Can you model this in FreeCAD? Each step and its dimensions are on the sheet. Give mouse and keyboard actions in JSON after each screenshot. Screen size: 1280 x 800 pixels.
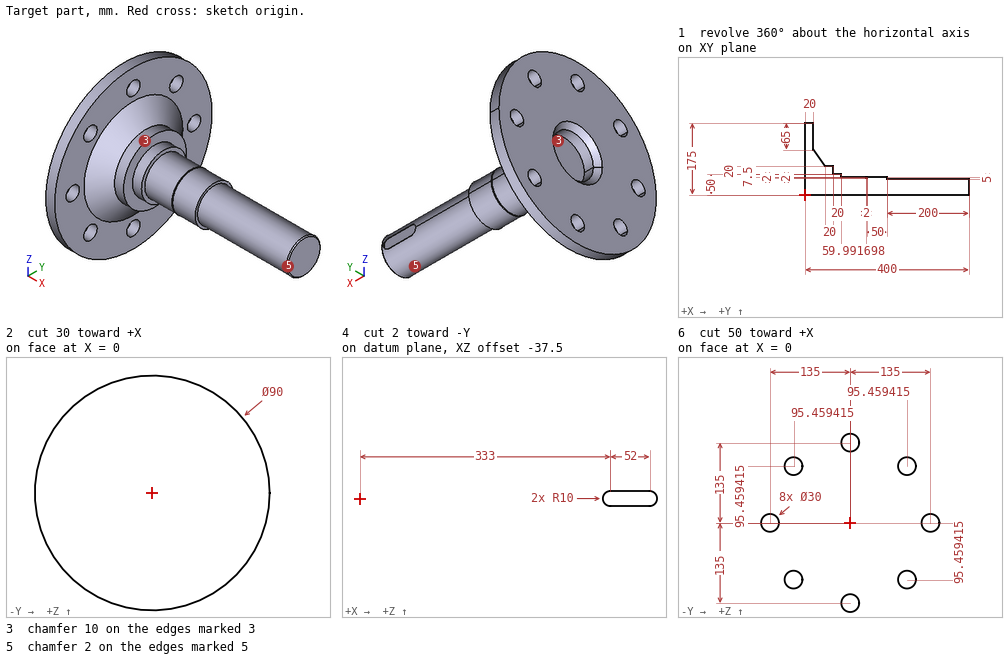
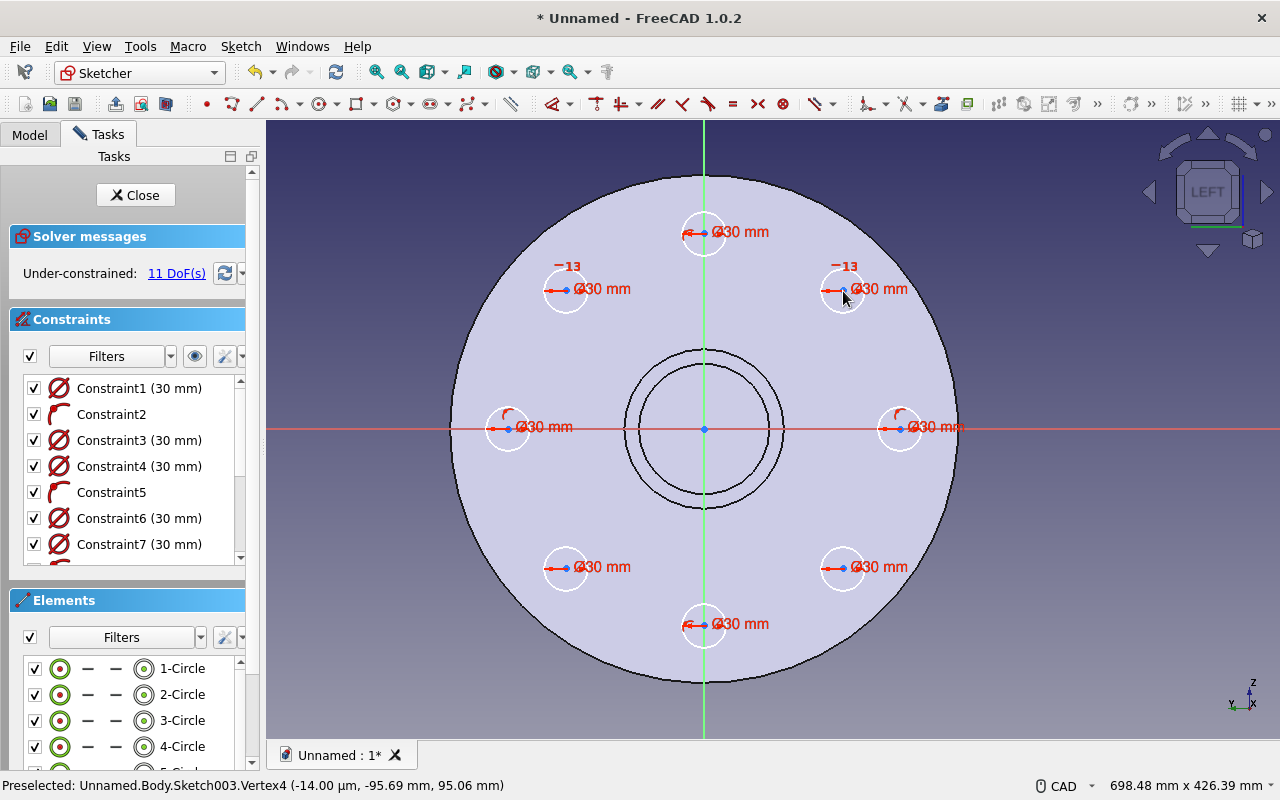
{"action": "left_click", "coordinate": [843, 291]}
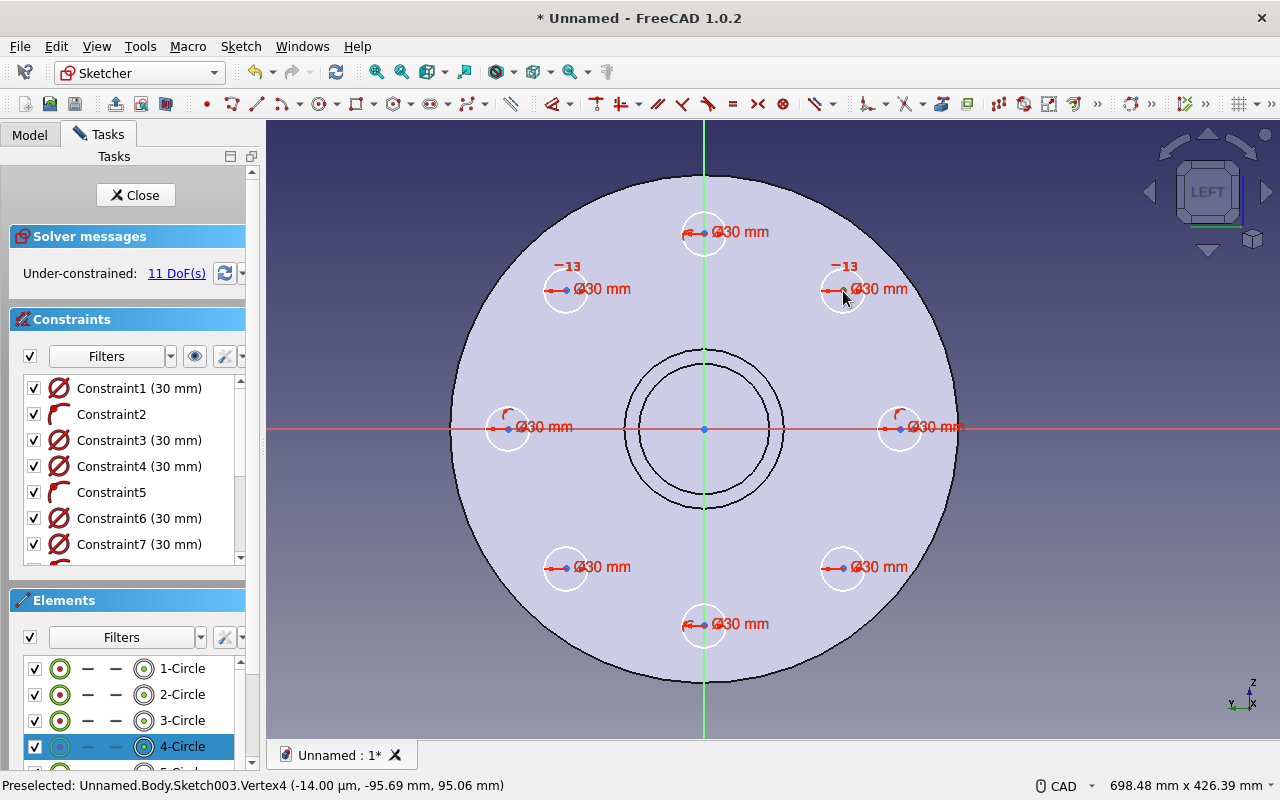
{"action": "left_click", "coordinate": [843, 569]}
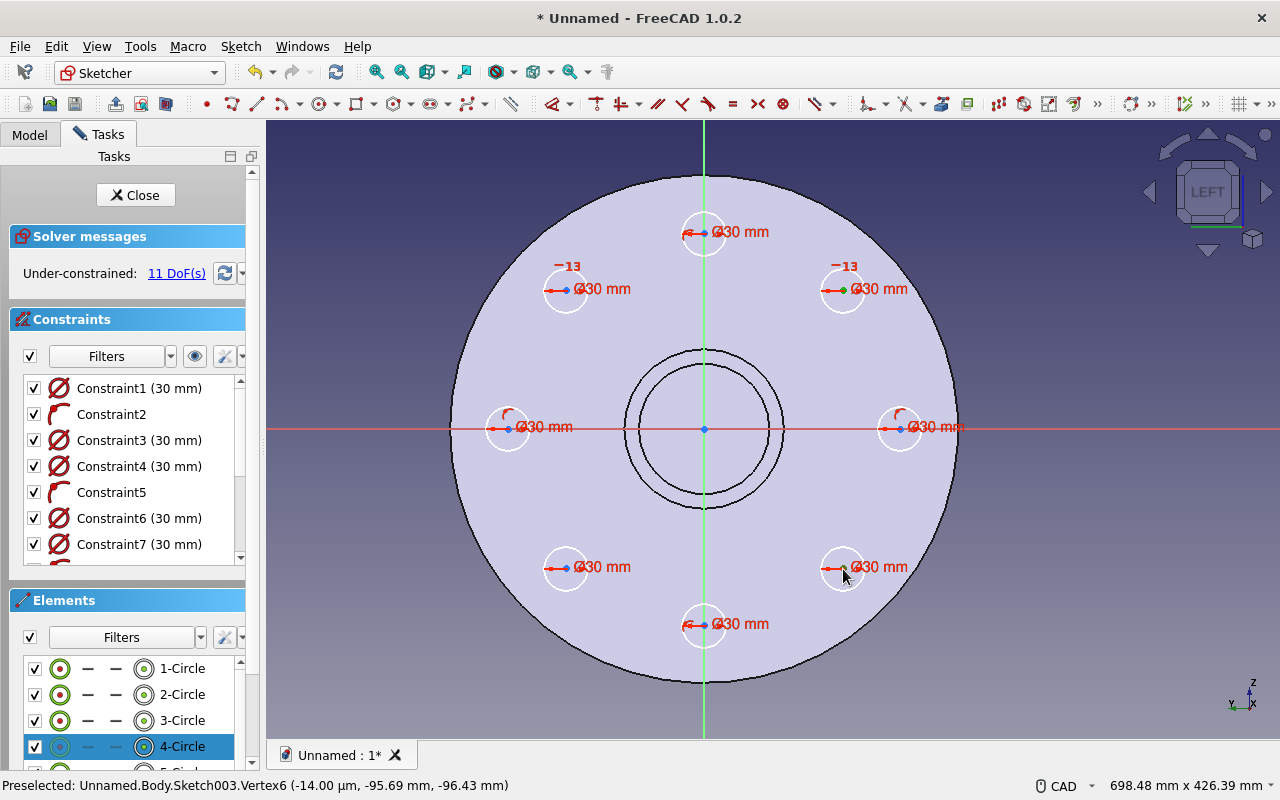
{"action": "key", "text": "v"}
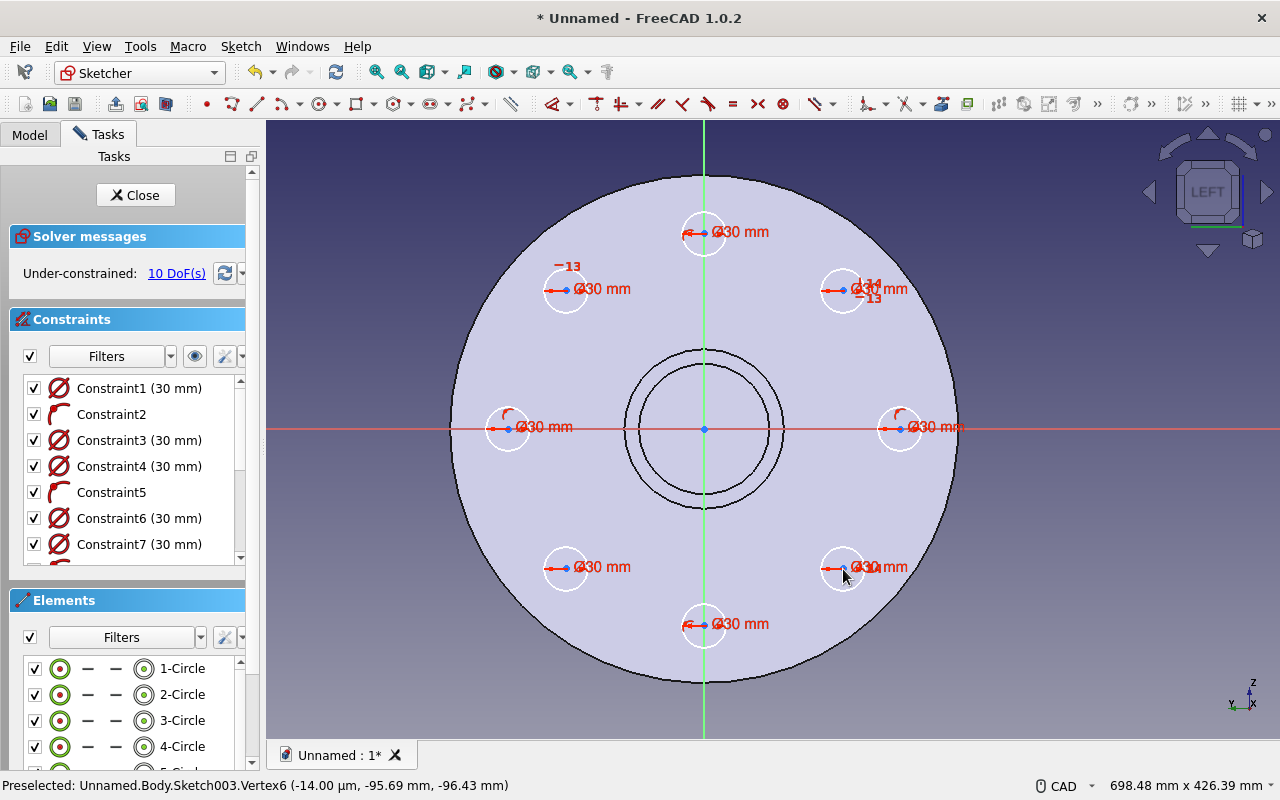
{"action": "left_click", "coordinate": [566, 291]}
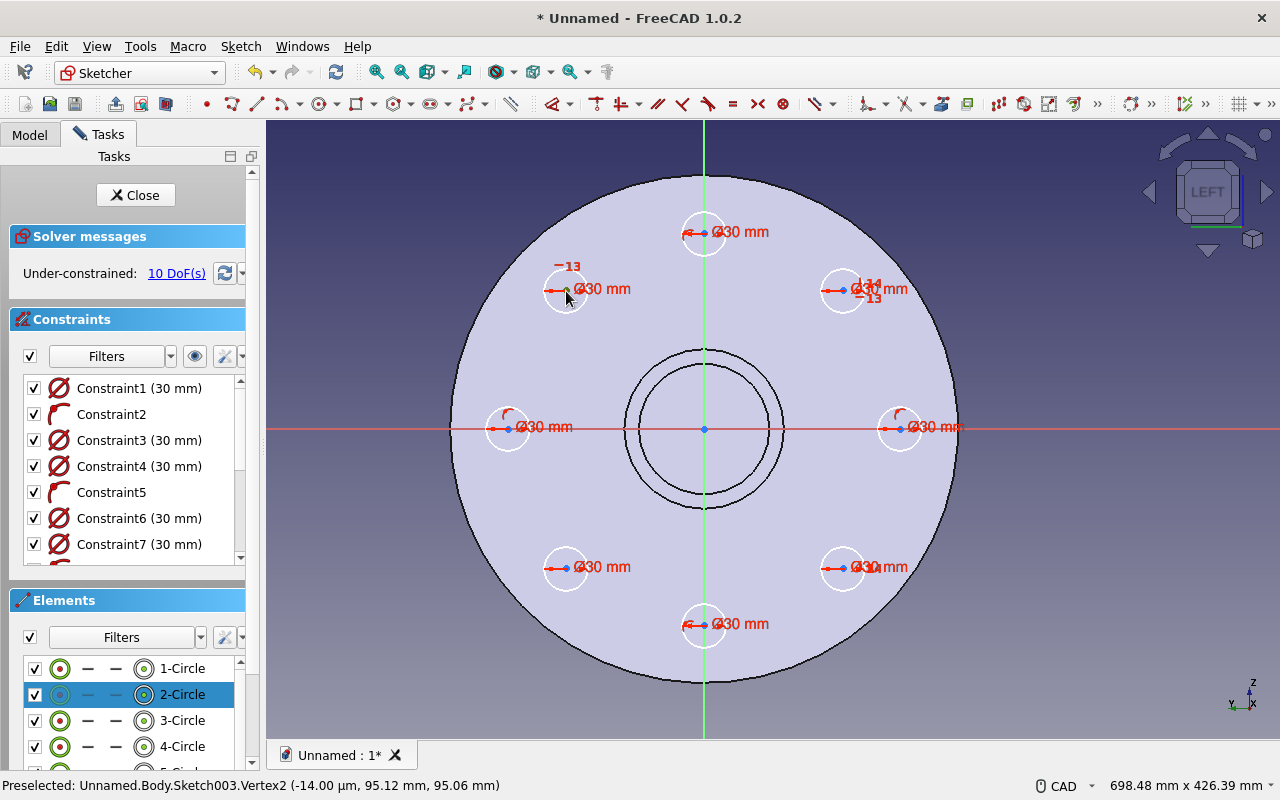
{"action": "left_click", "coordinate": [566, 569]}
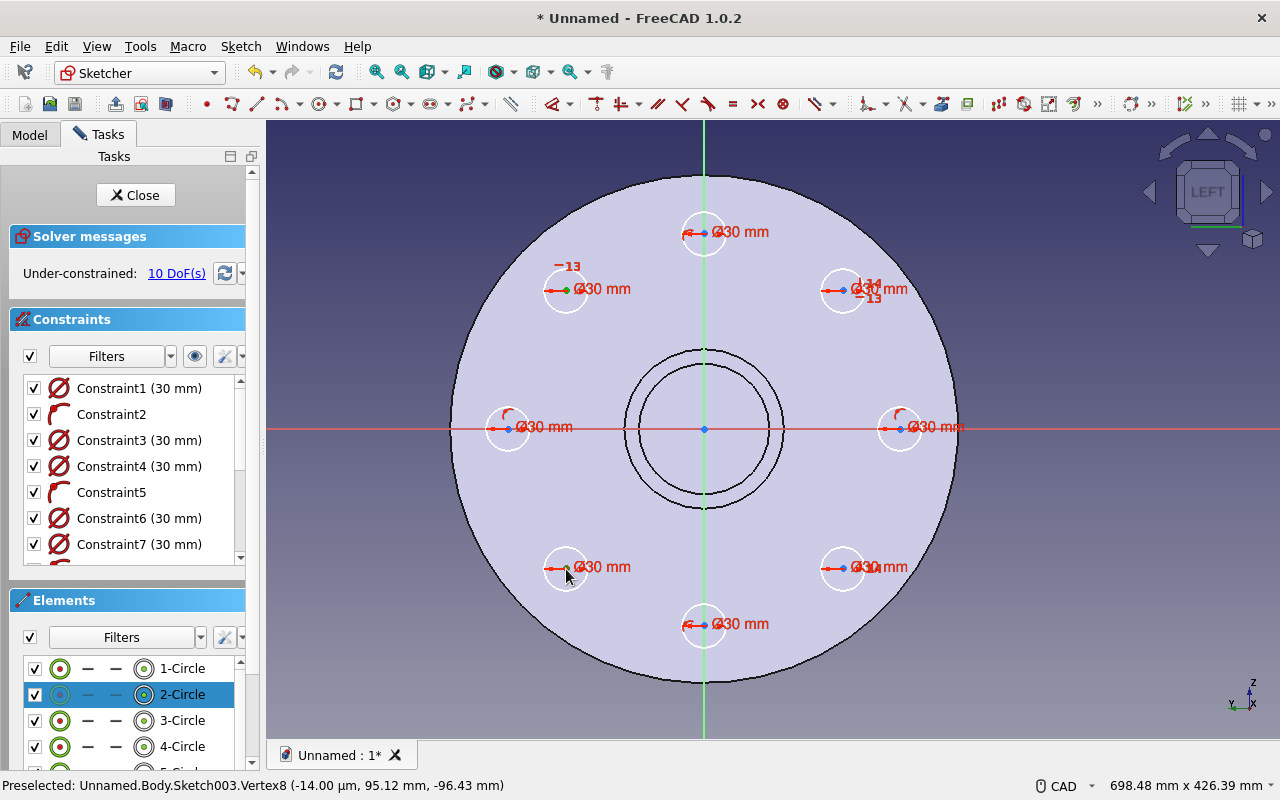
{"action": "key", "text": "v"}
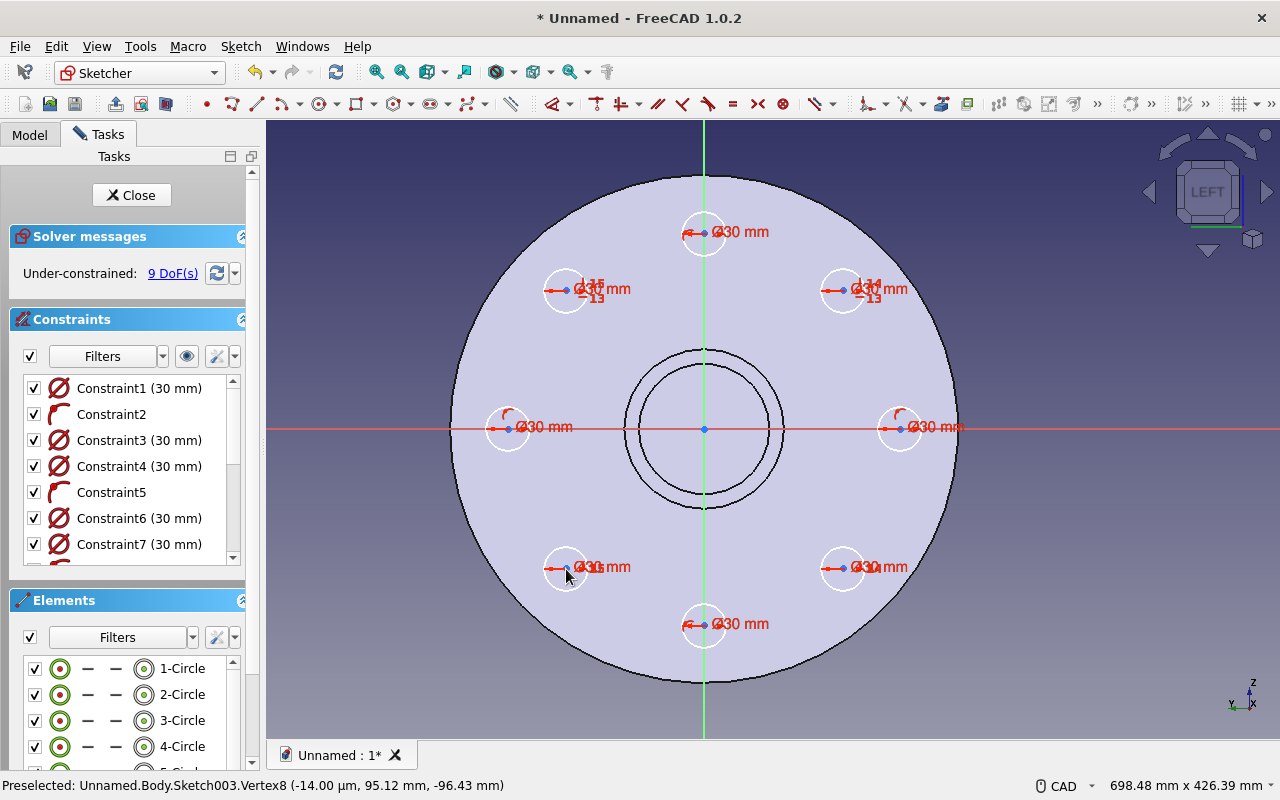
{"action": "left_click", "coordinate": [843, 569]}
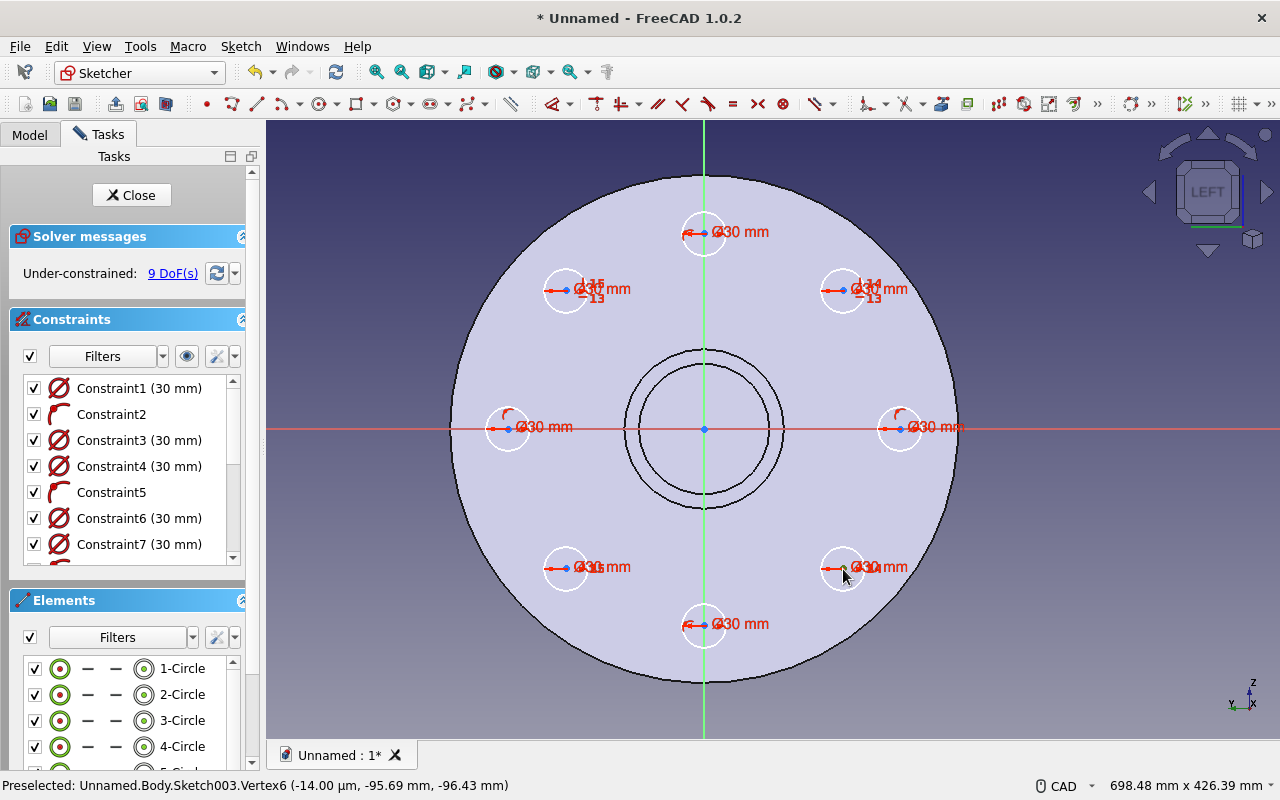
{"action": "left_click", "coordinate": [566, 569]}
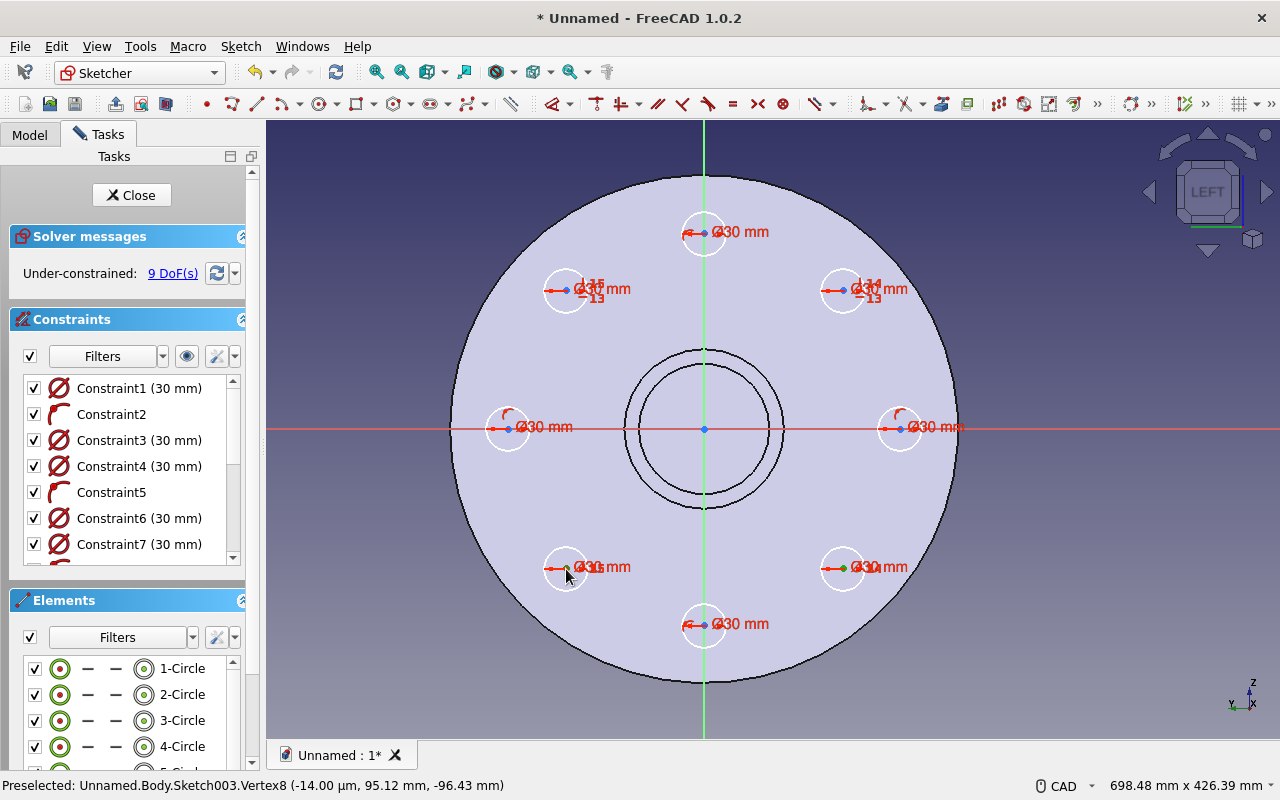
{"action": "key", "text": "h"}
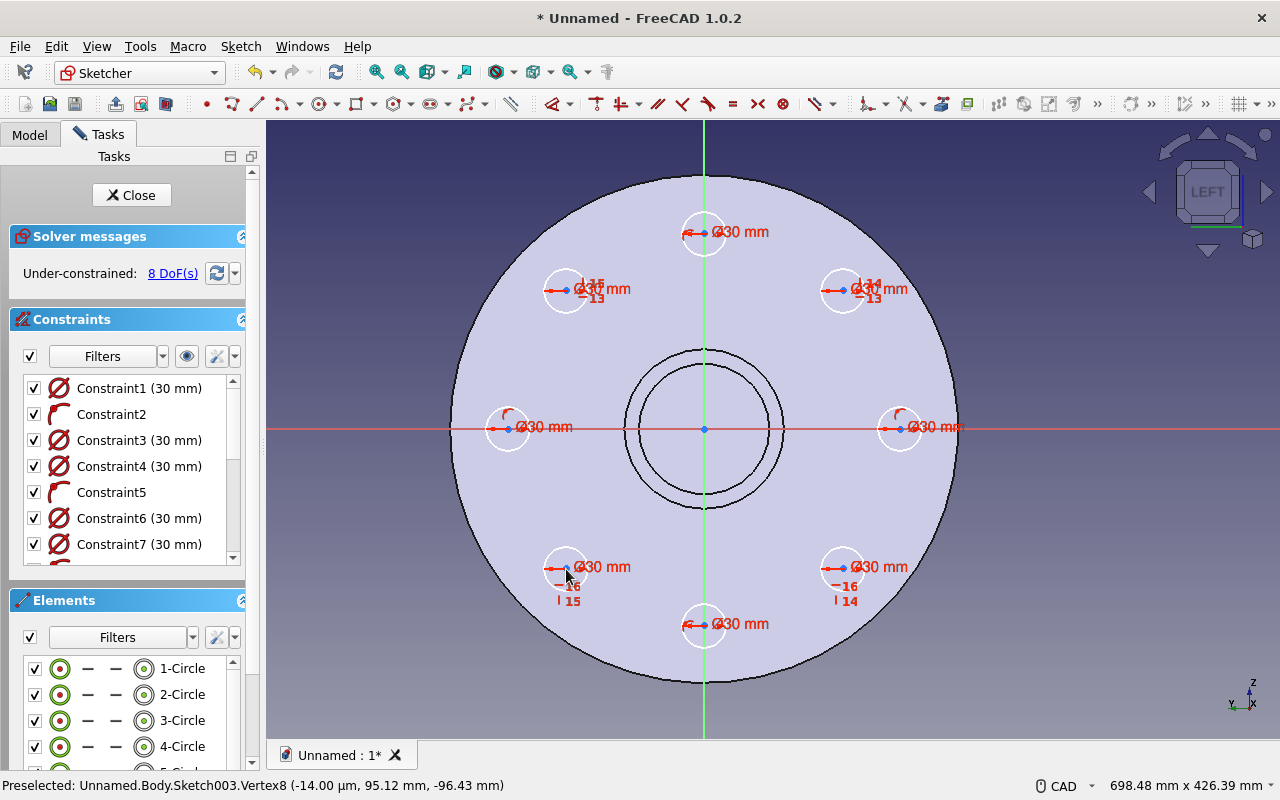
{"action": "left_click", "coordinate": [552, 104]}